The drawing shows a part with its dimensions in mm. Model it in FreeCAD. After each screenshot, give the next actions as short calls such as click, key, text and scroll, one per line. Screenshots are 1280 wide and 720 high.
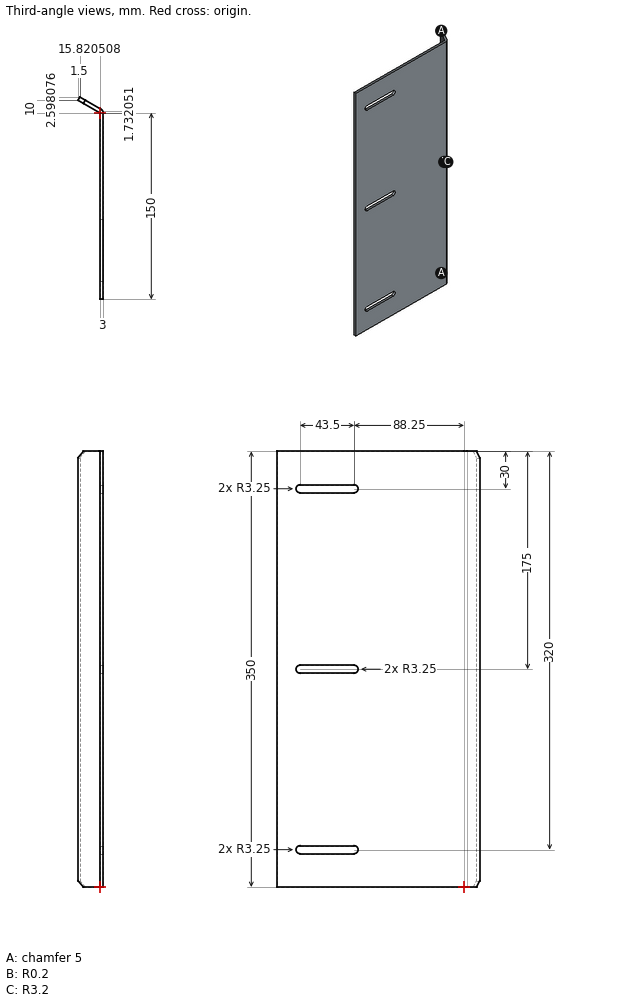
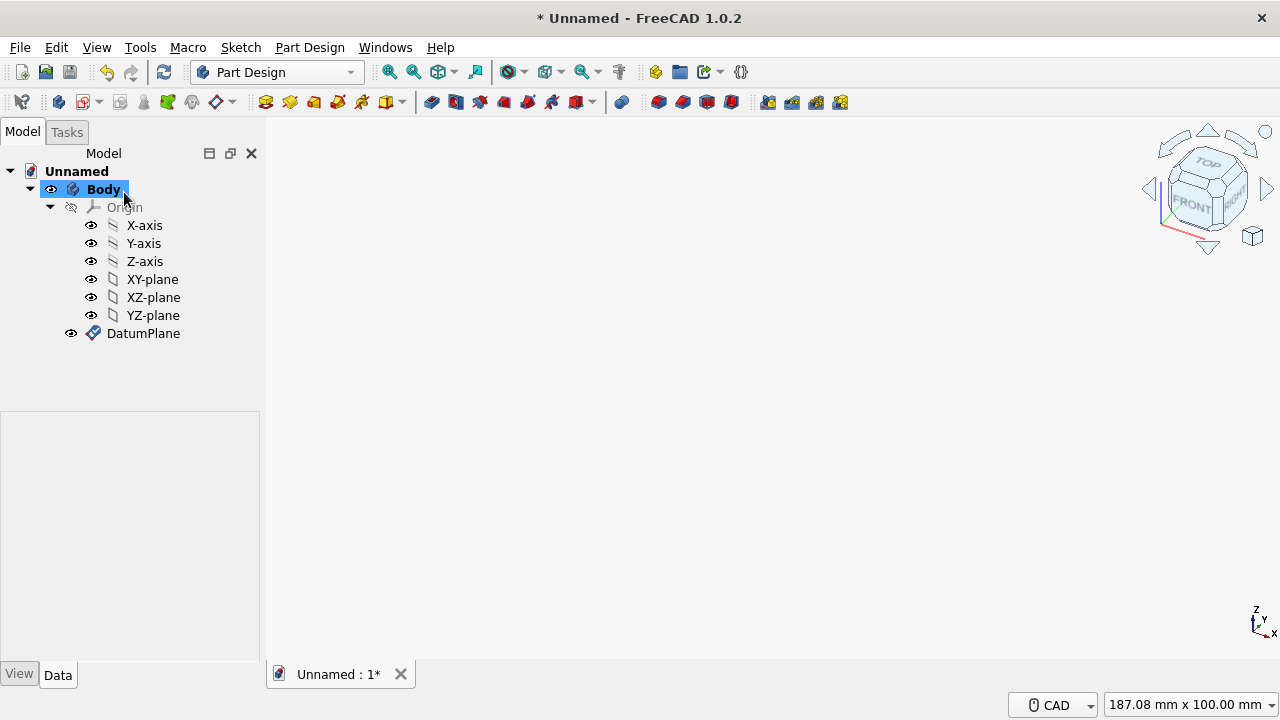
click(116, 333)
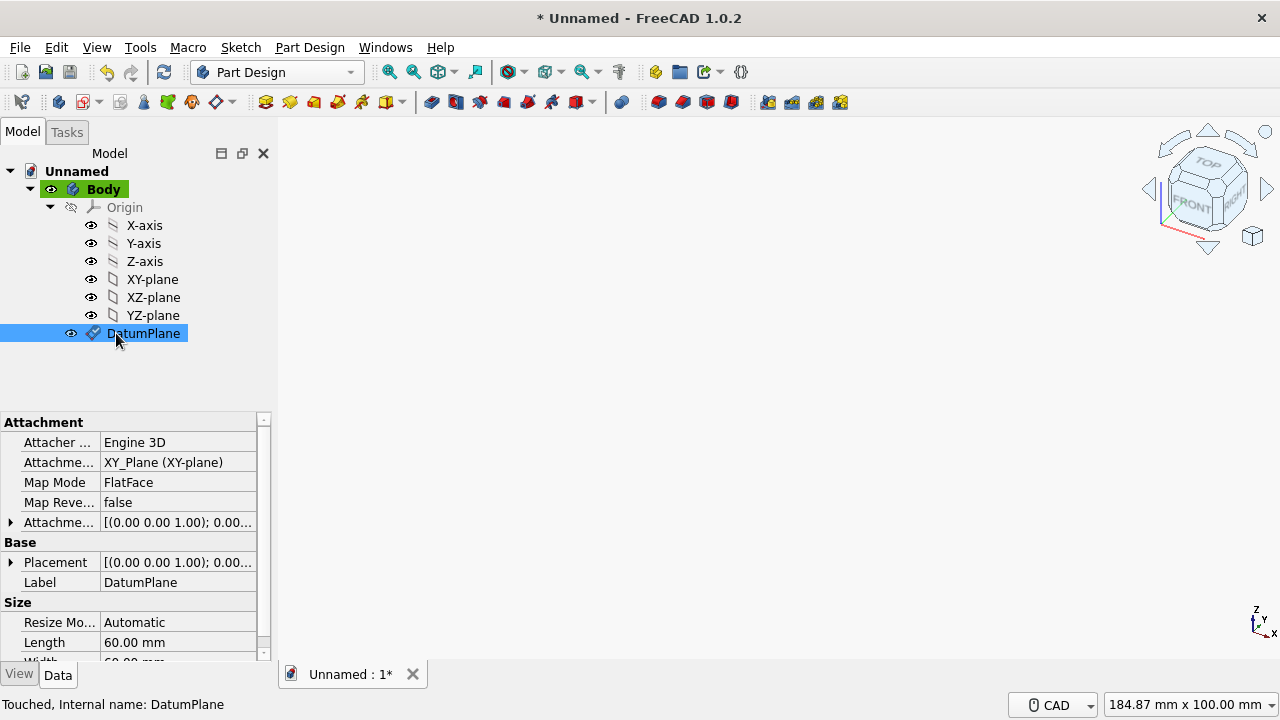
click(84, 102)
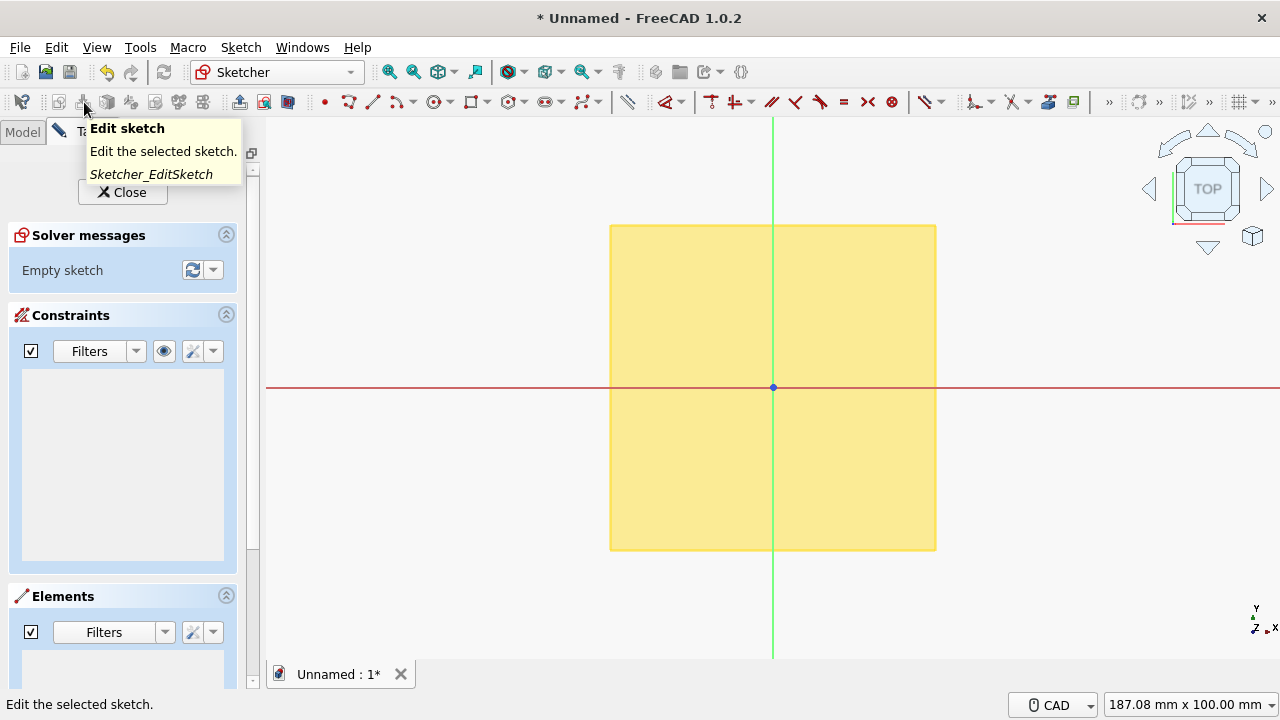
scroll(687, 171, down, 5)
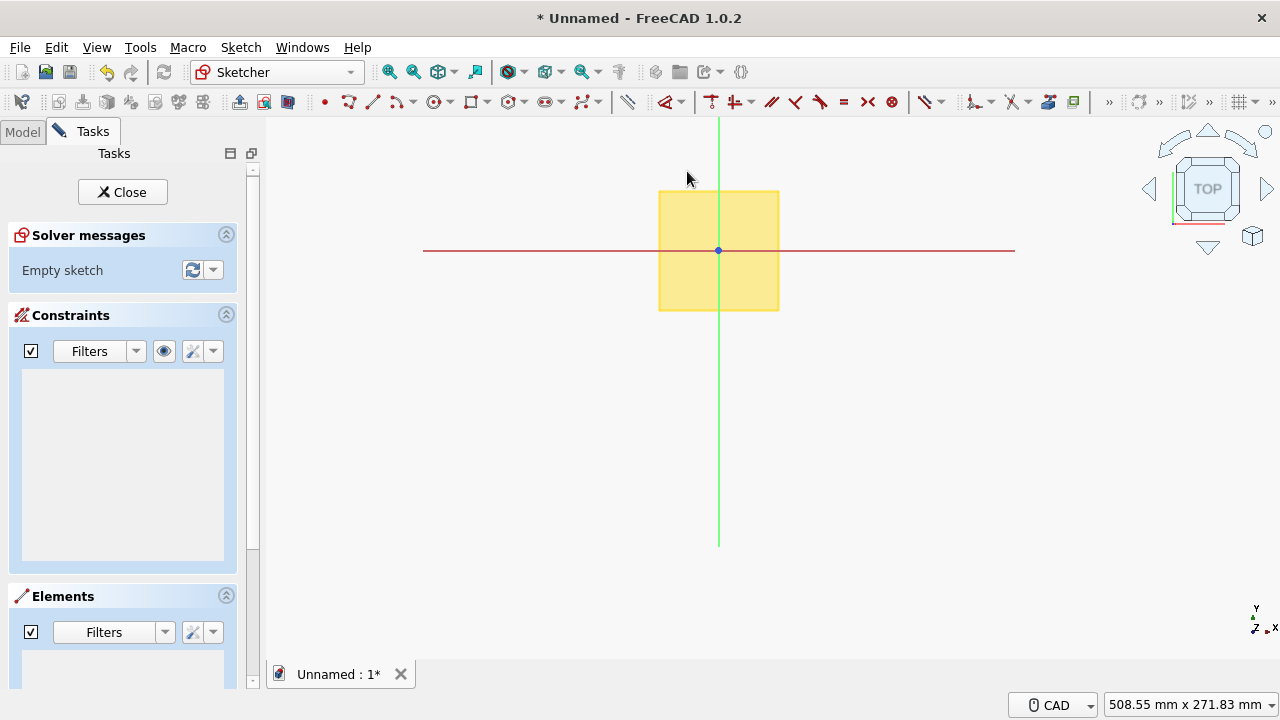
click(350, 102)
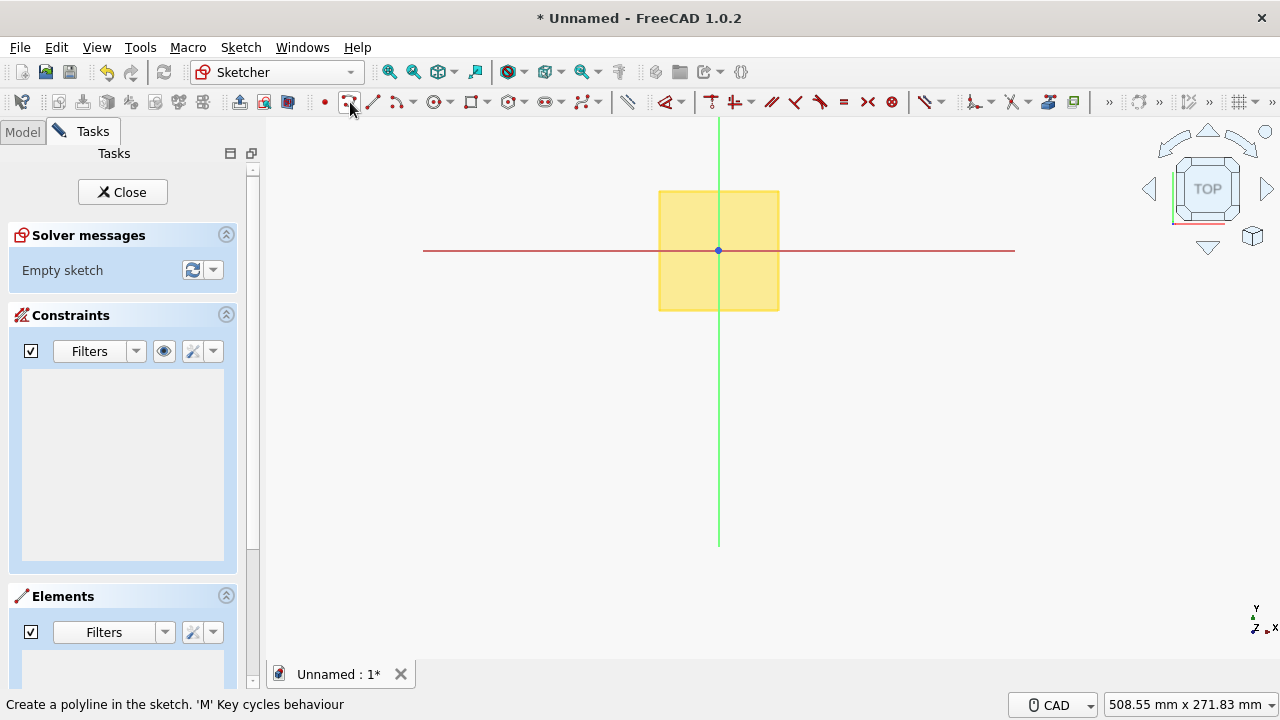
click(719, 251)
click(710, 550)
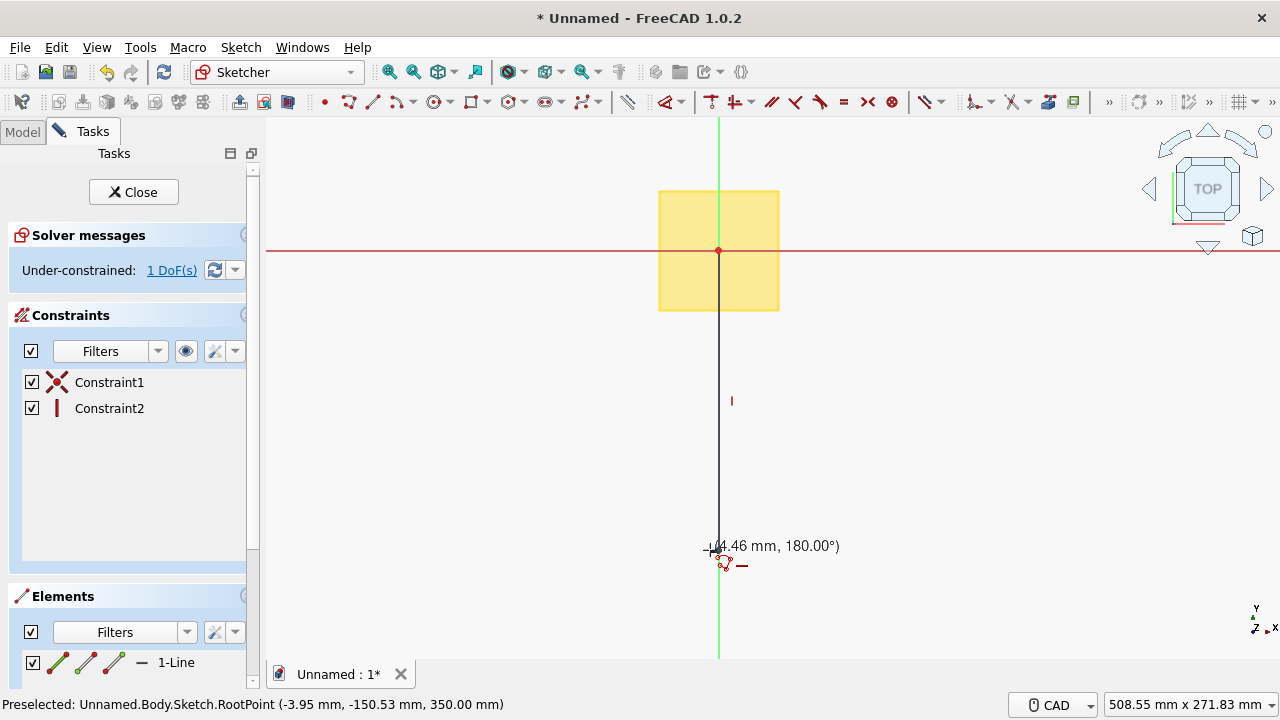
scroll(725, 550, up, 5)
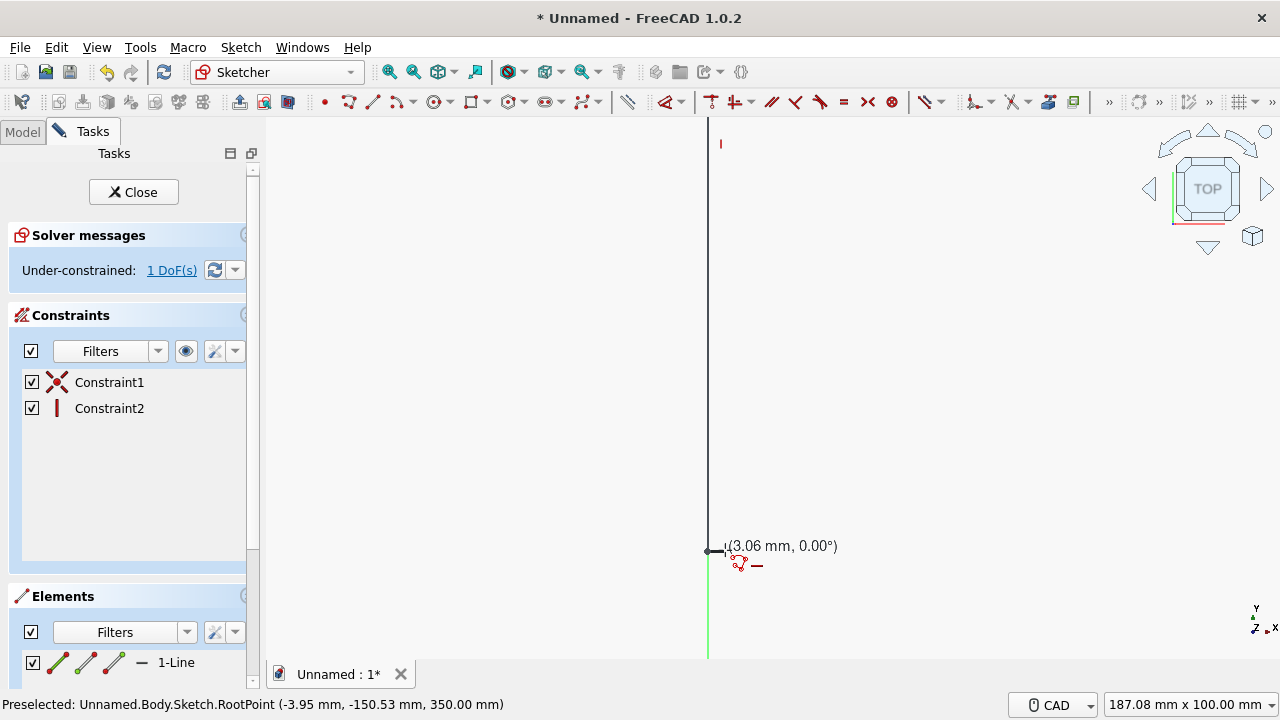
click(724, 549)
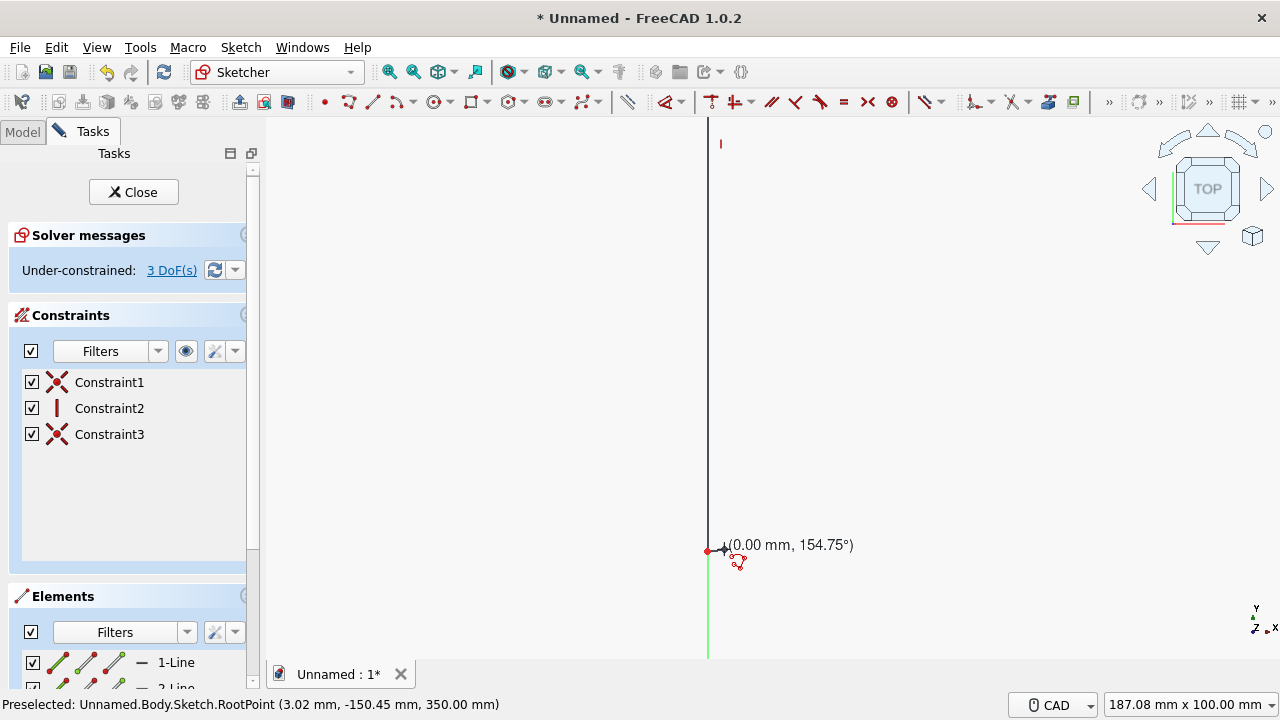
scroll(725, 551, down, 5)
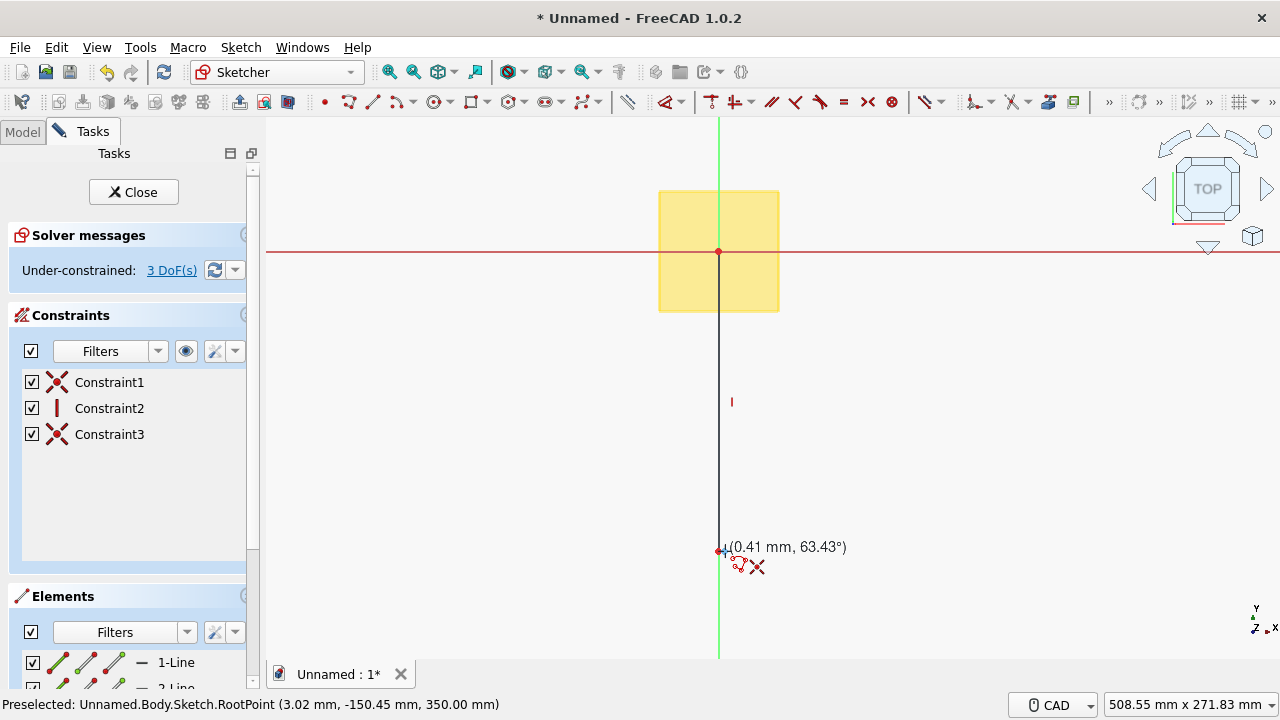
scroll(725, 248, up, 8)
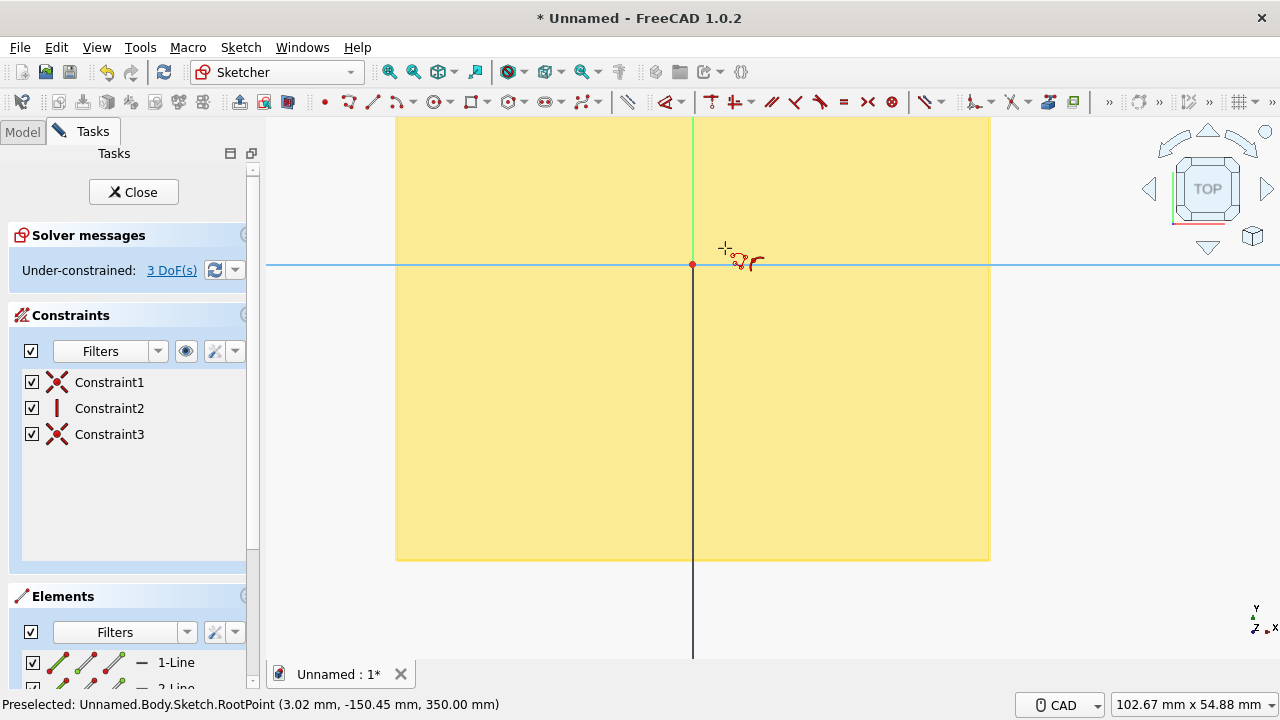
click(723, 247)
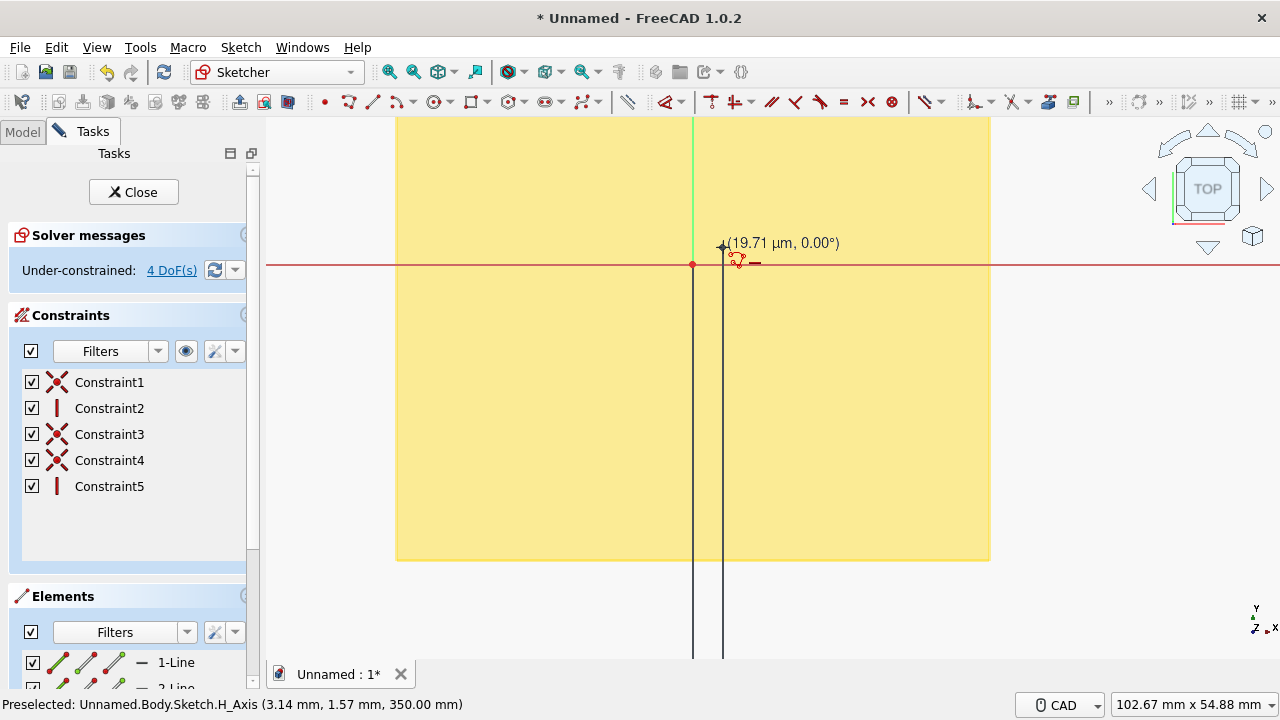
scroll(725, 248, down, 8)